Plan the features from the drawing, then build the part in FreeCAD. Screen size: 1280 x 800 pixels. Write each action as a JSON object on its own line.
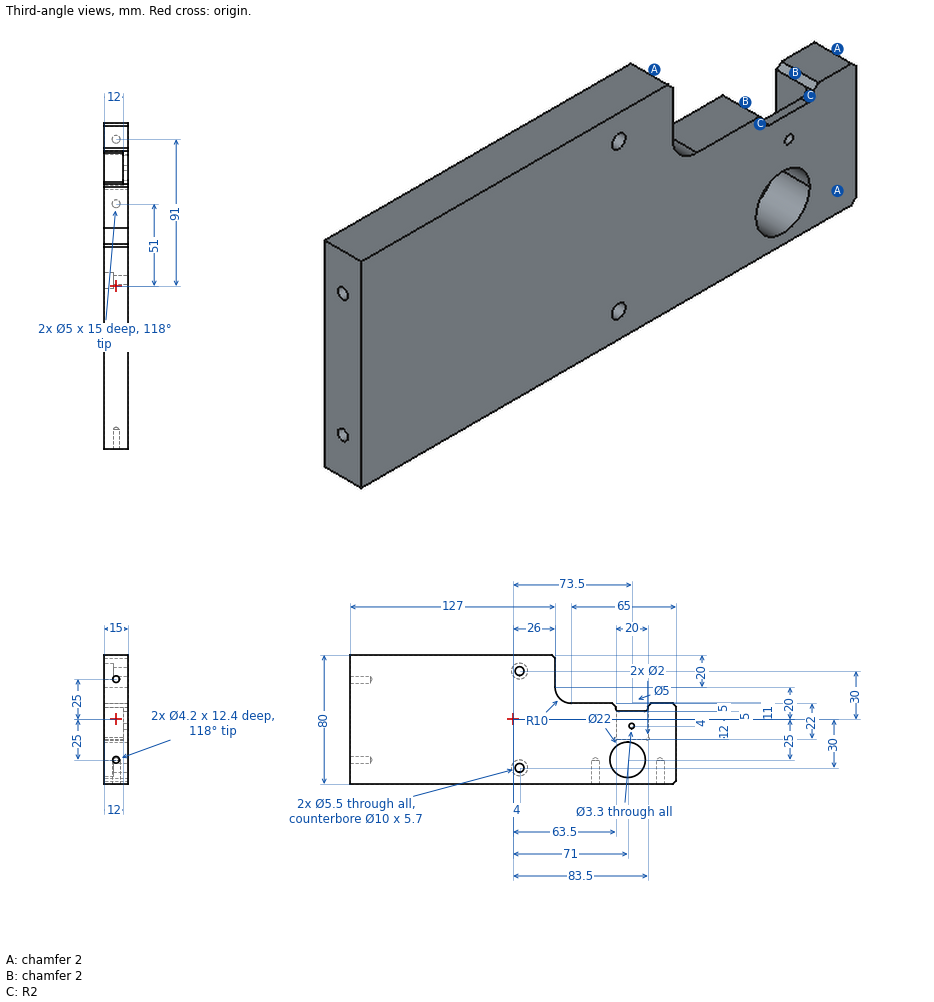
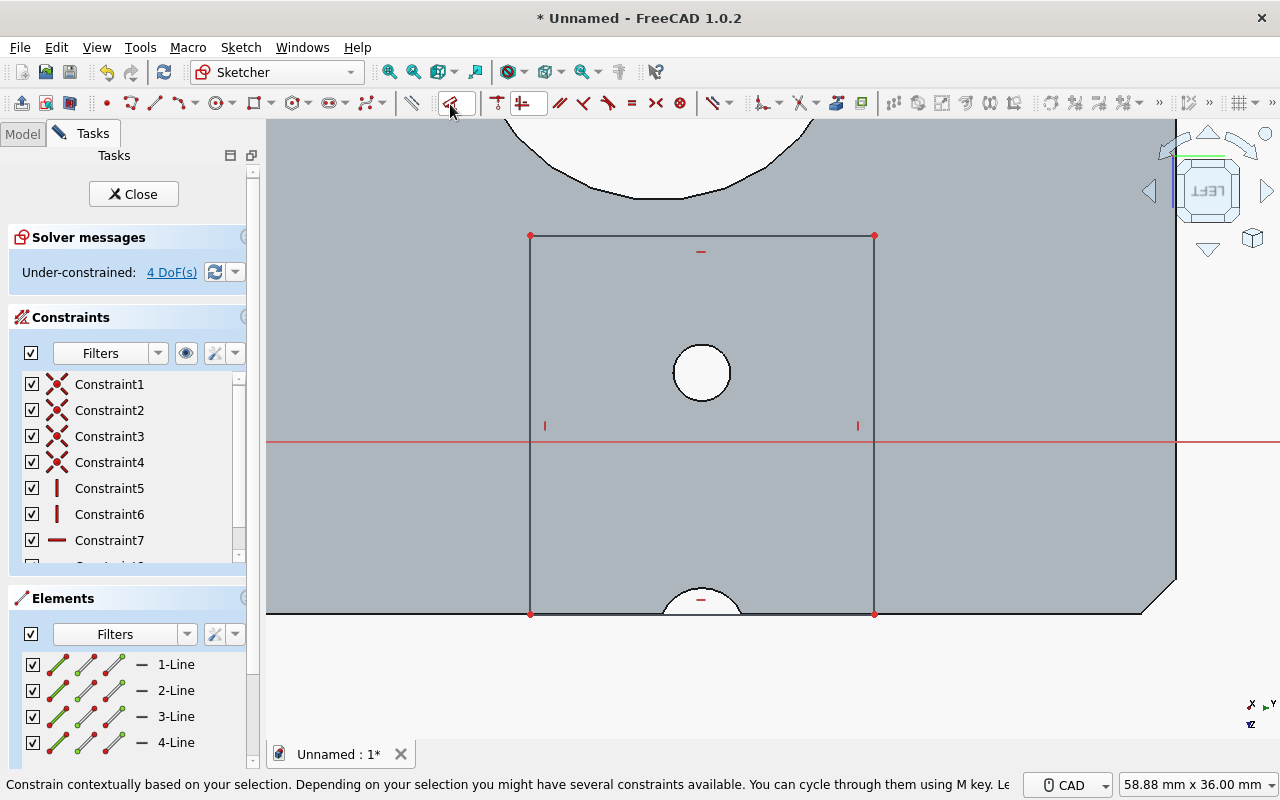
{"action": "left_click", "coordinate": [530, 350]}
{"action": "left_click", "coordinate": [496, 426]}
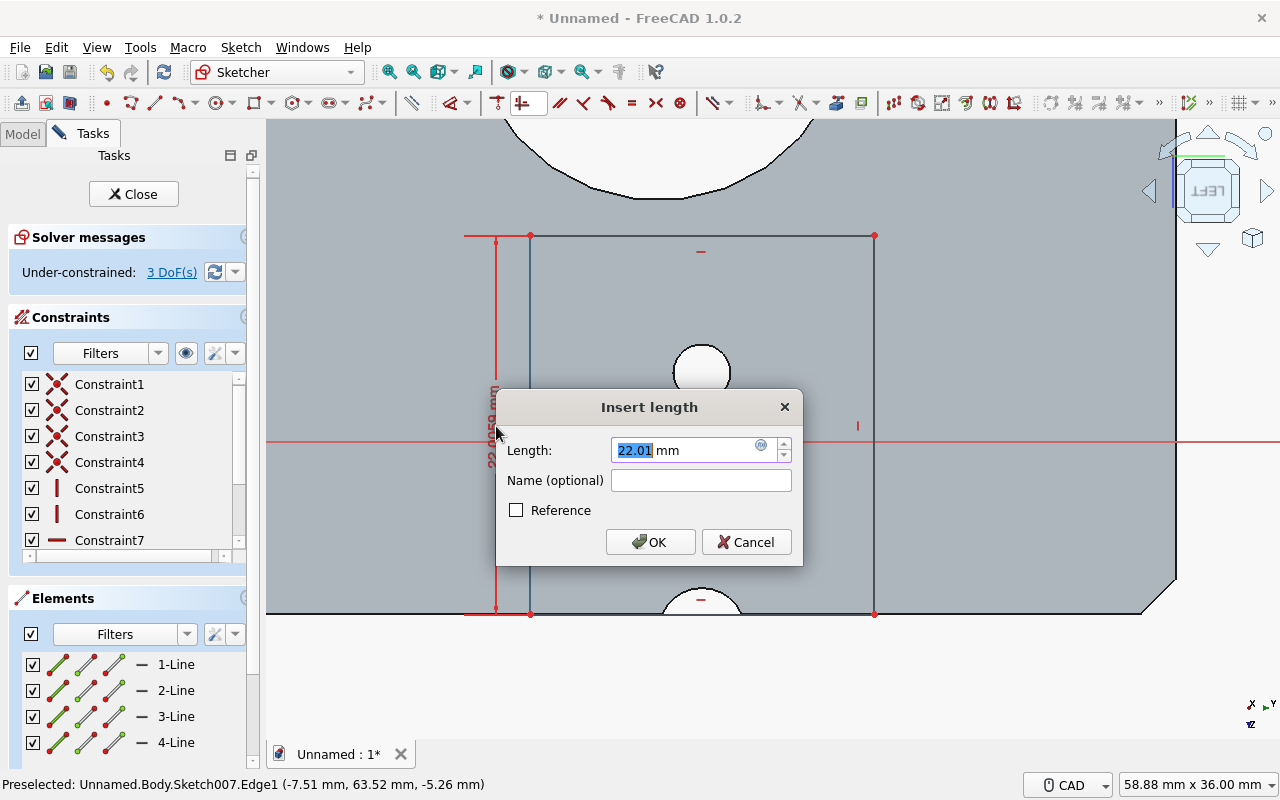
{"action": "type", "text": "22"}
{"action": "key", "text": "Return"}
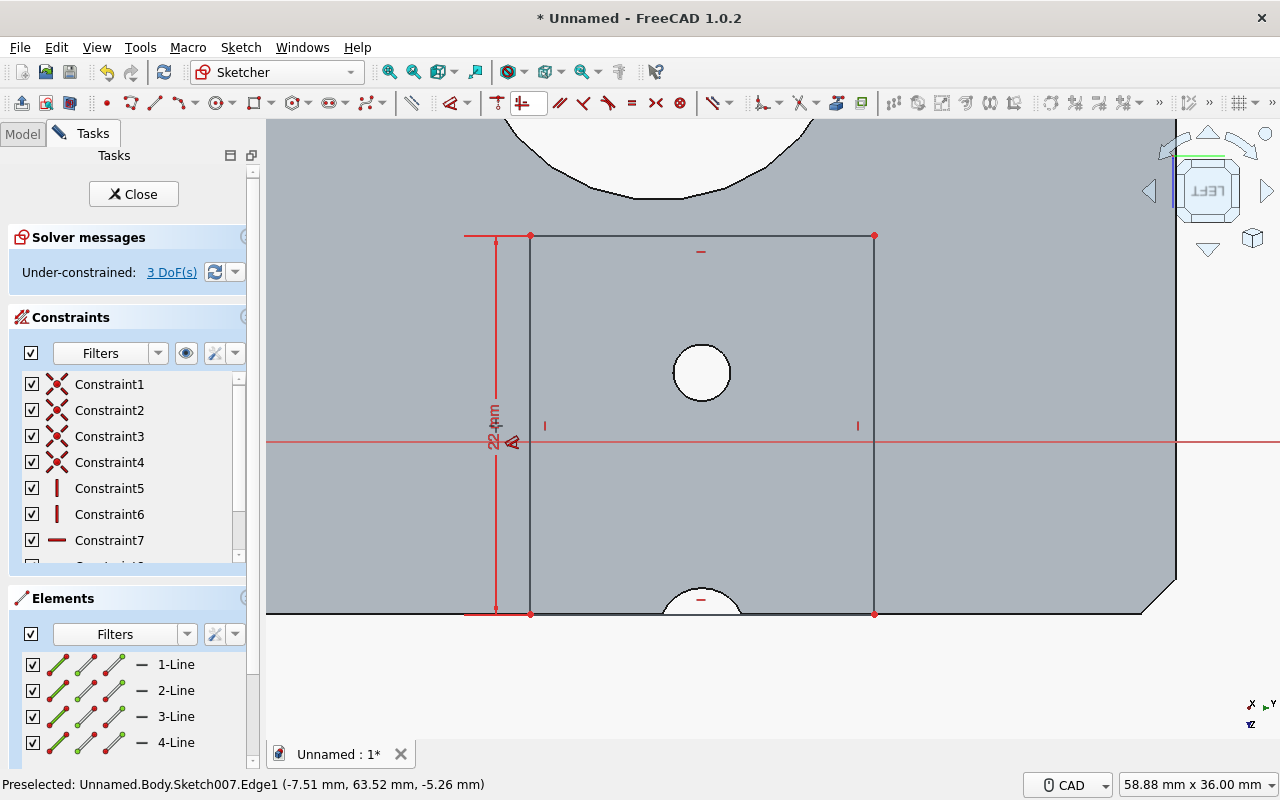
{"action": "left_click", "coordinate": [633, 615]}
{"action": "left_click", "coordinate": [702, 649]}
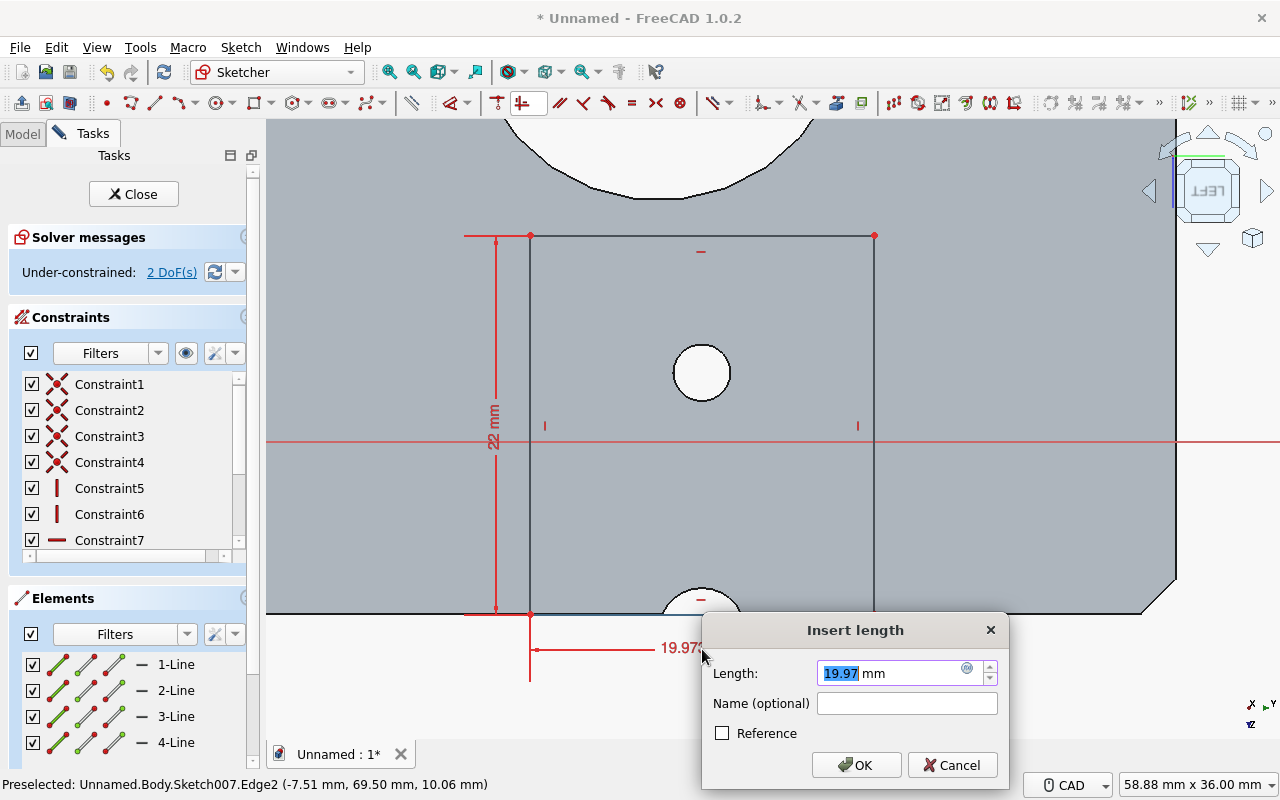
{"action": "type", "text": "20"}
{"action": "key", "text": "Return"}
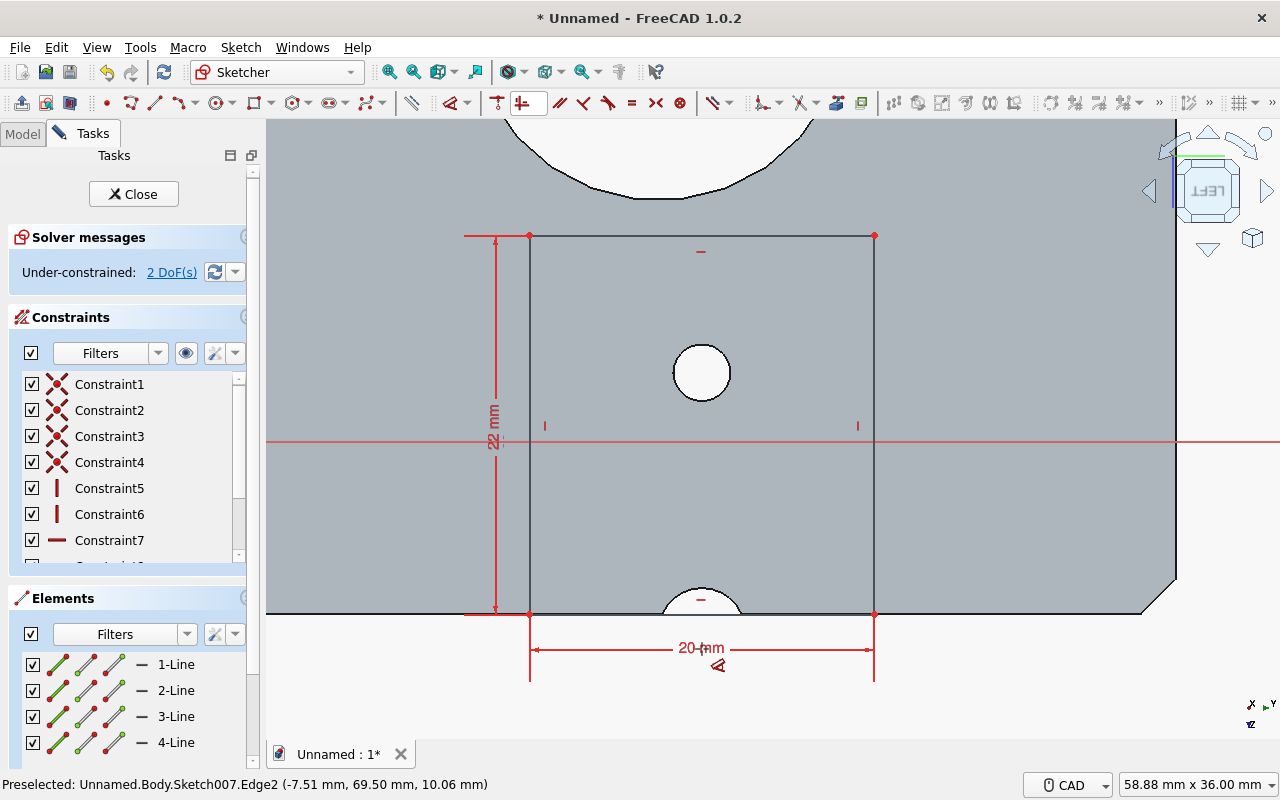
{"action": "left_click", "coordinate": [530, 236]}
{"action": "left_click", "coordinate": [564, 339]}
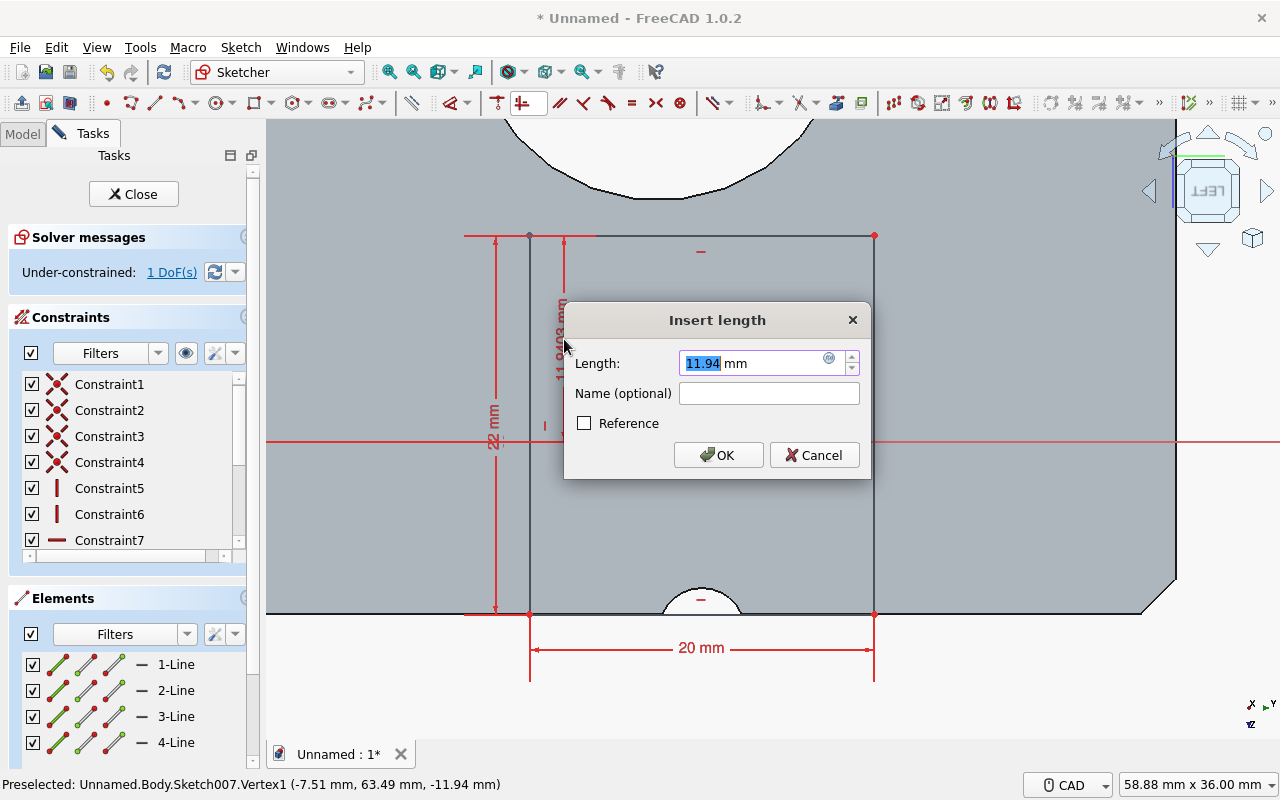
{"action": "type", "text": "12"}
{"action": "key", "text": "Return"}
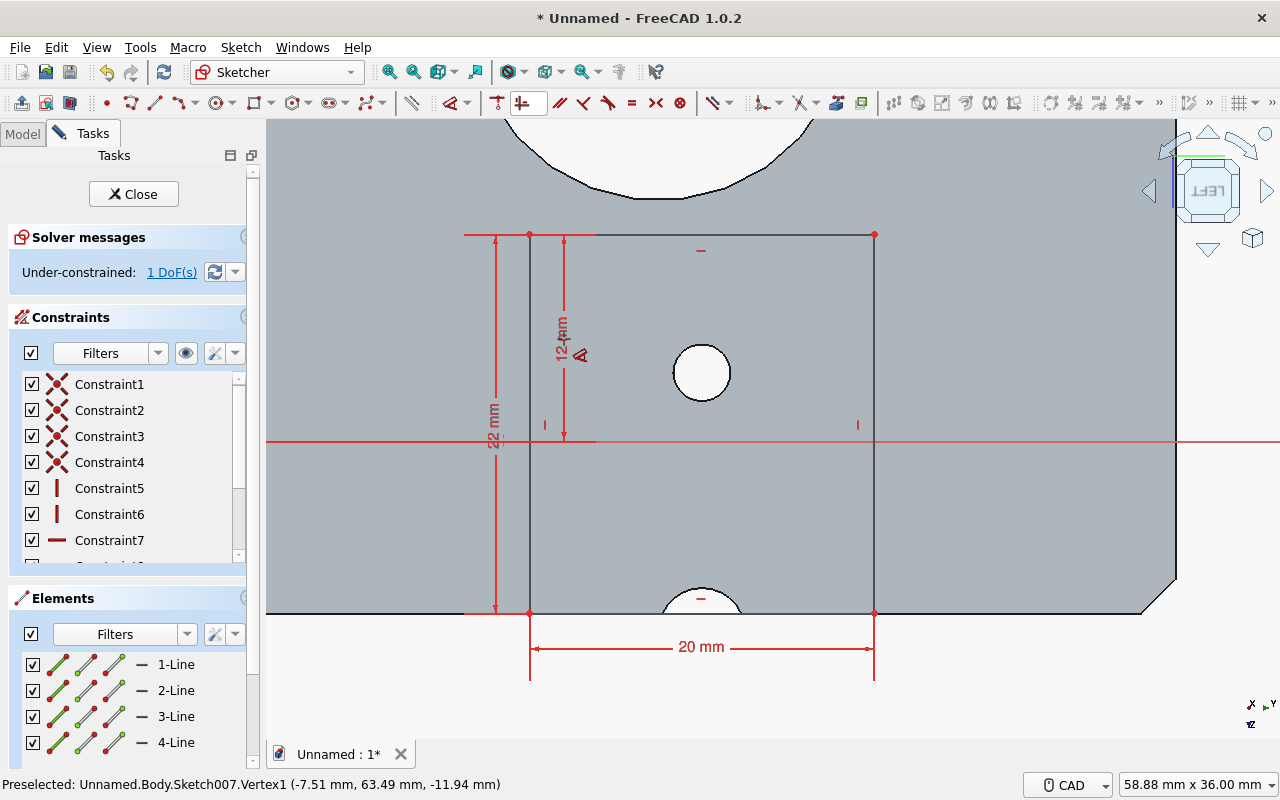
{"action": "left_click", "coordinate": [530, 235]}
{"action": "left_click", "coordinate": [412, 201]}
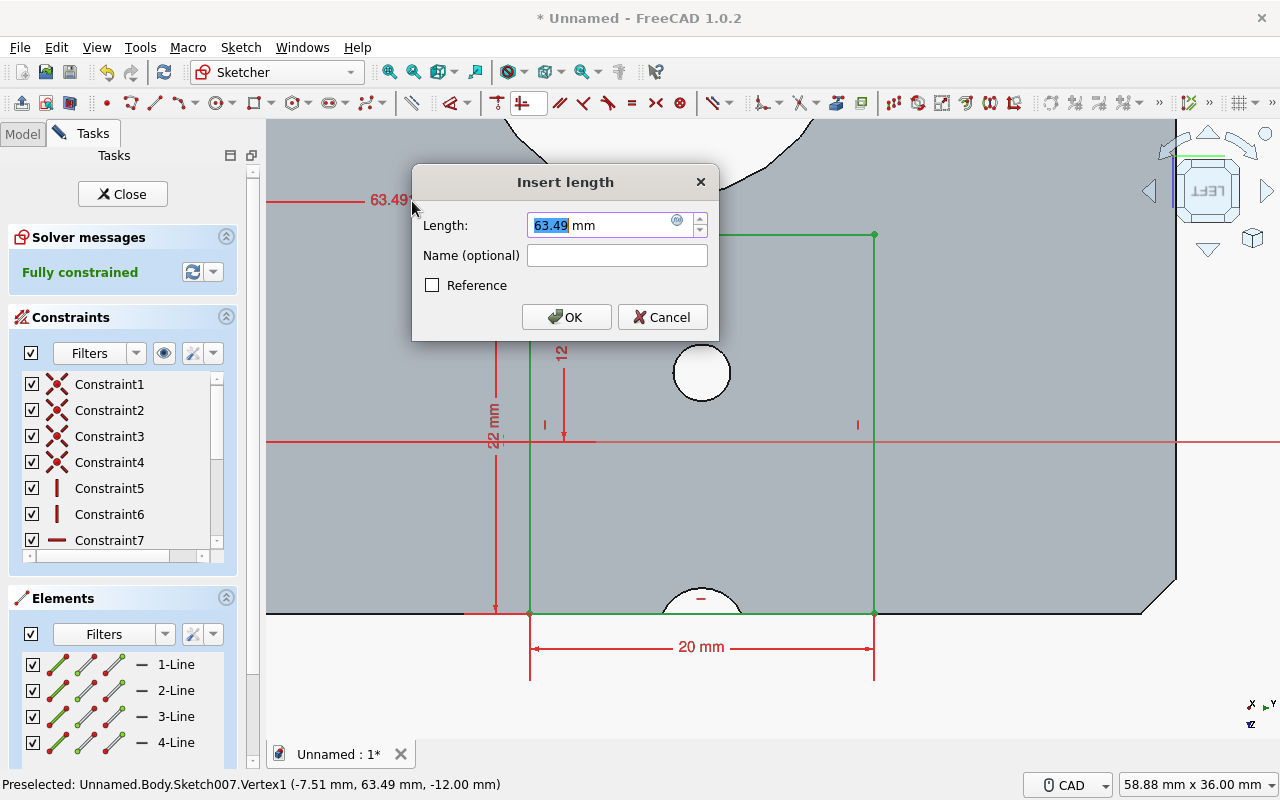
{"action": "type", "text": "63.5"}
{"action": "key", "text": "Return"}
{"action": "key", "text": "Escape"}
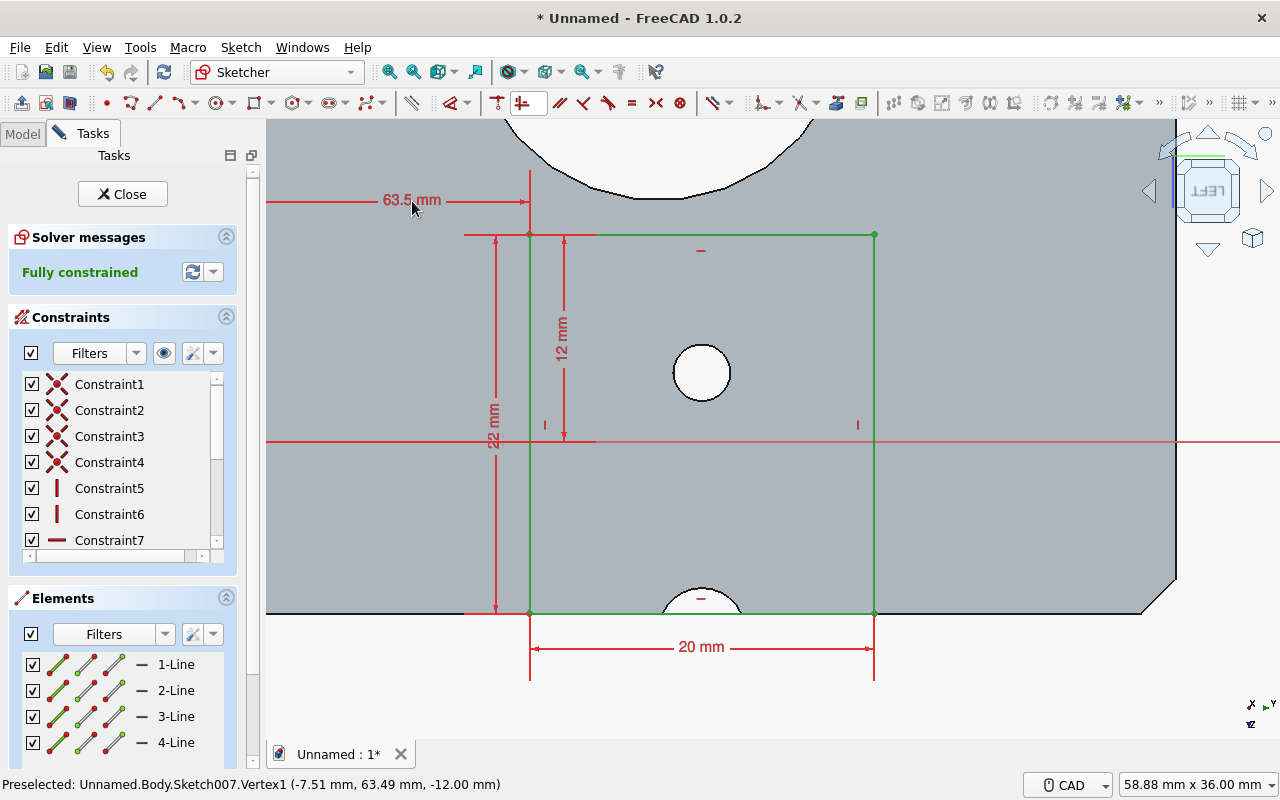
{"action": "left_click", "coordinate": [123, 194]}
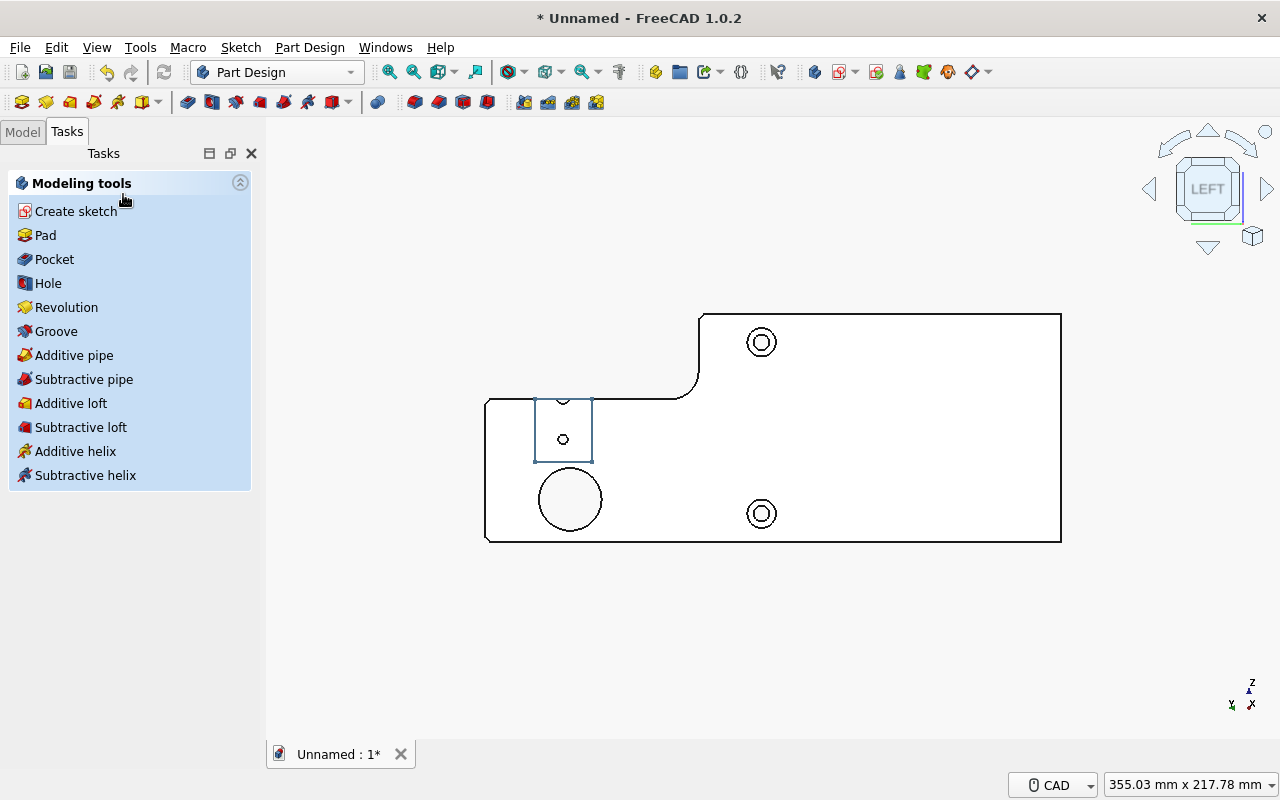
{"action": "left_click", "coordinate": [188, 102]}